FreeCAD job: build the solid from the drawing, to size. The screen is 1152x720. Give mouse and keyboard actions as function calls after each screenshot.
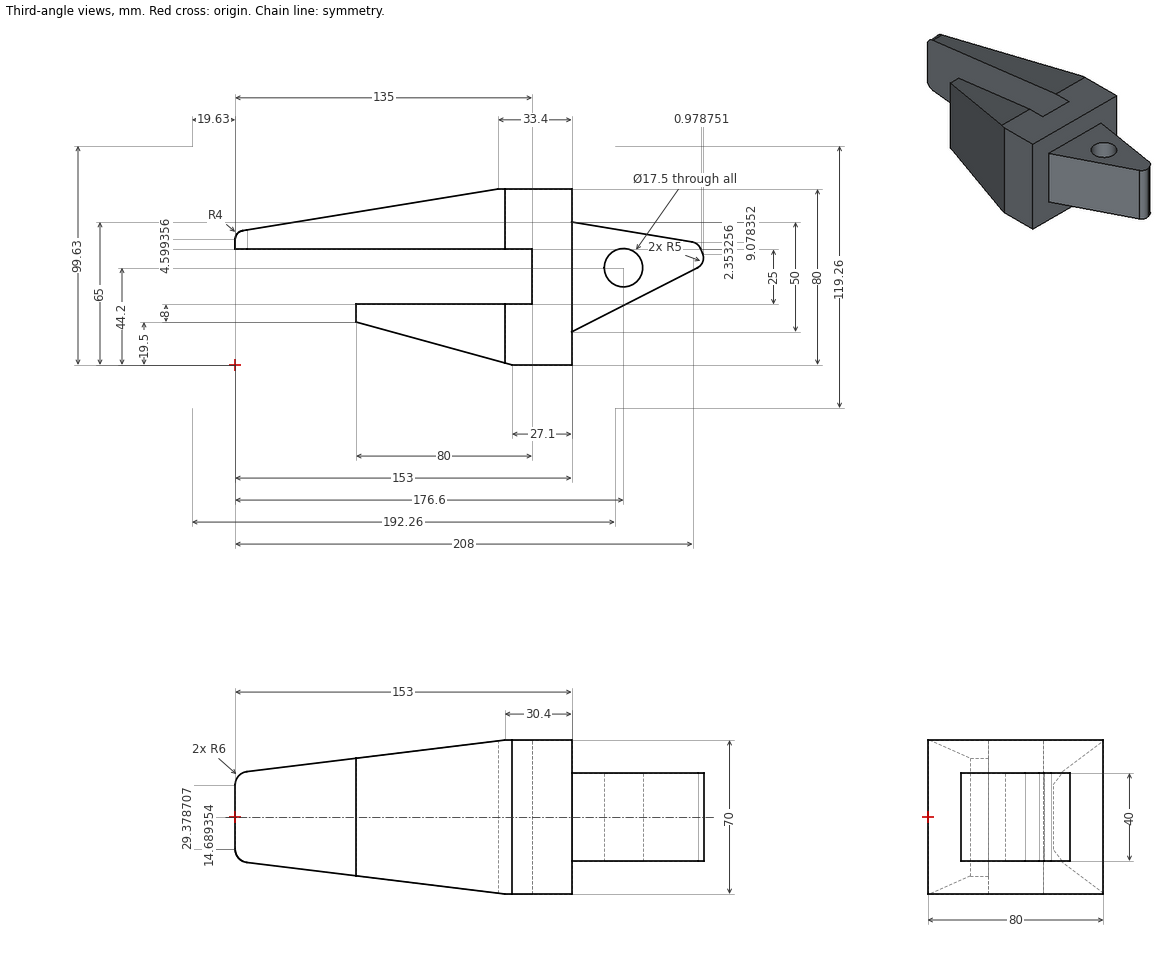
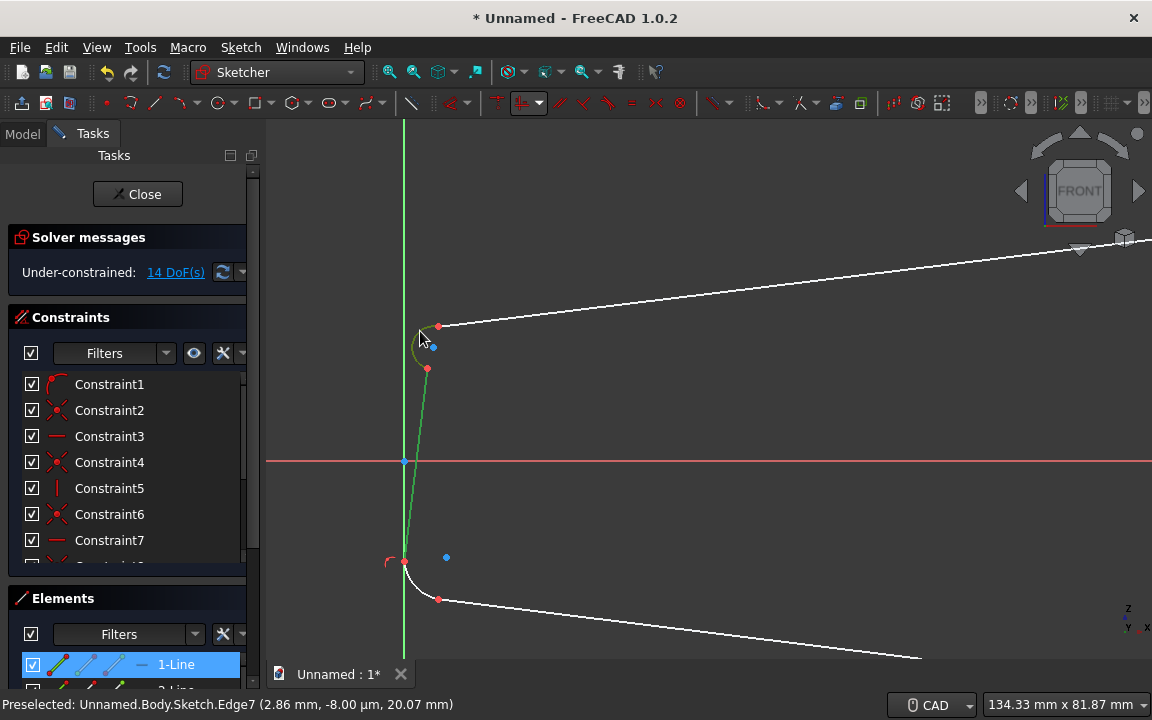
click(608, 104)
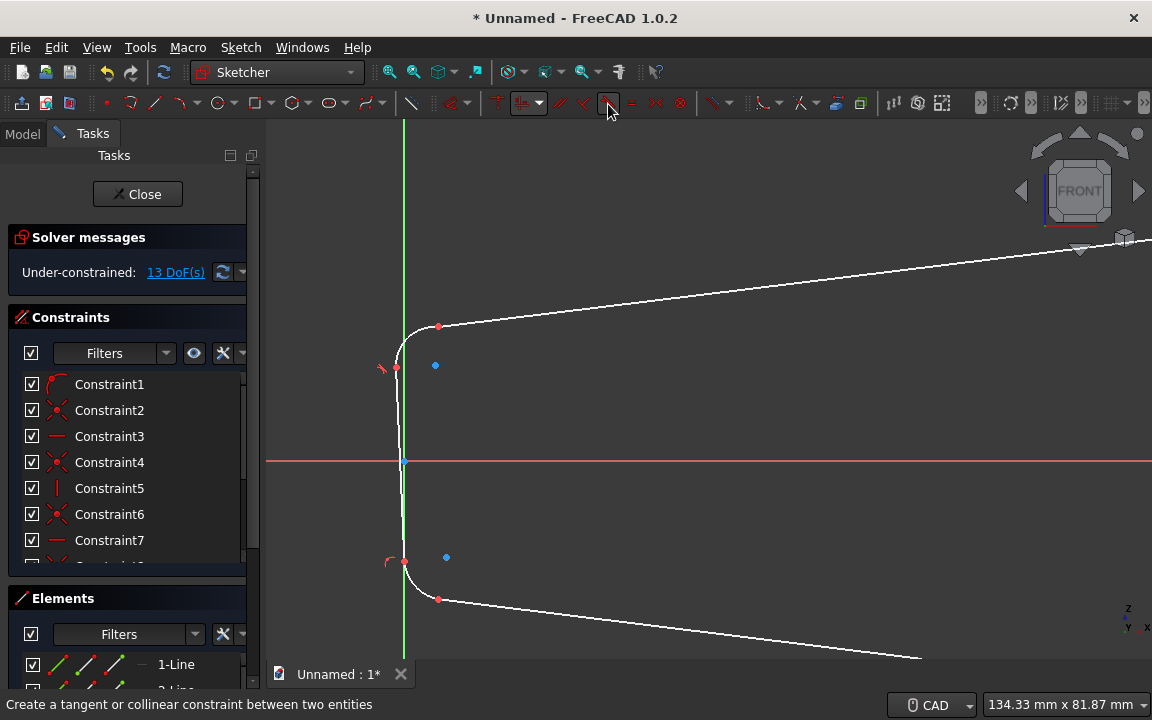
click(402, 503)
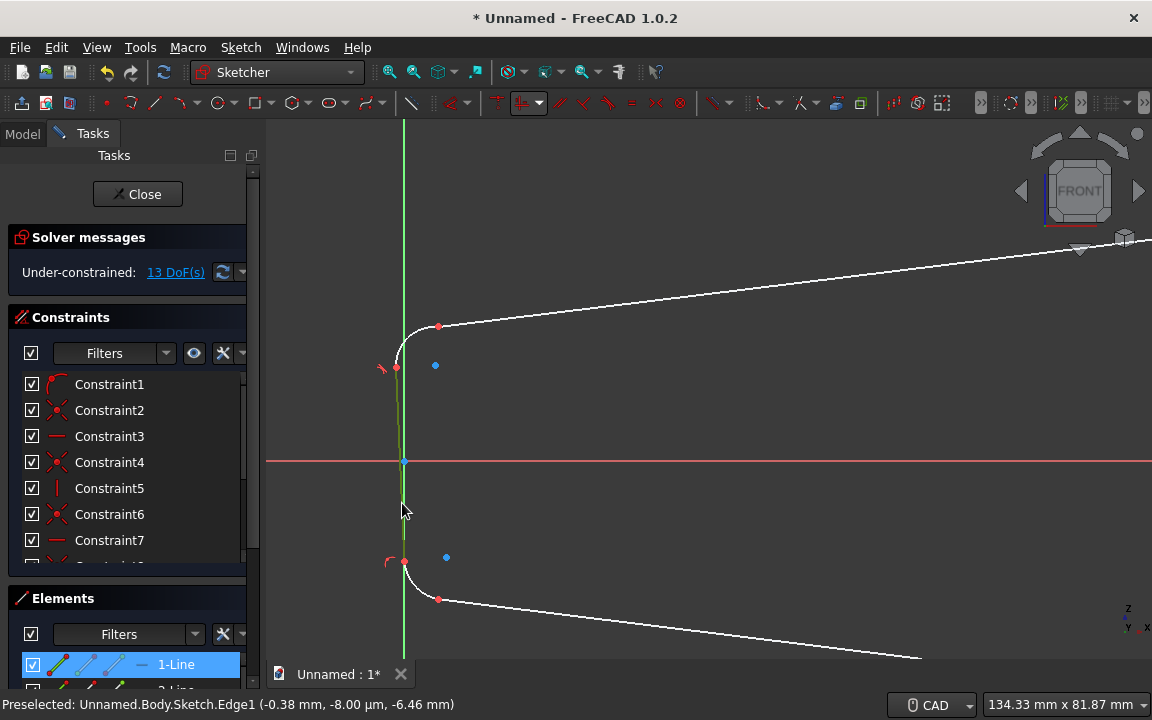
click(424, 593)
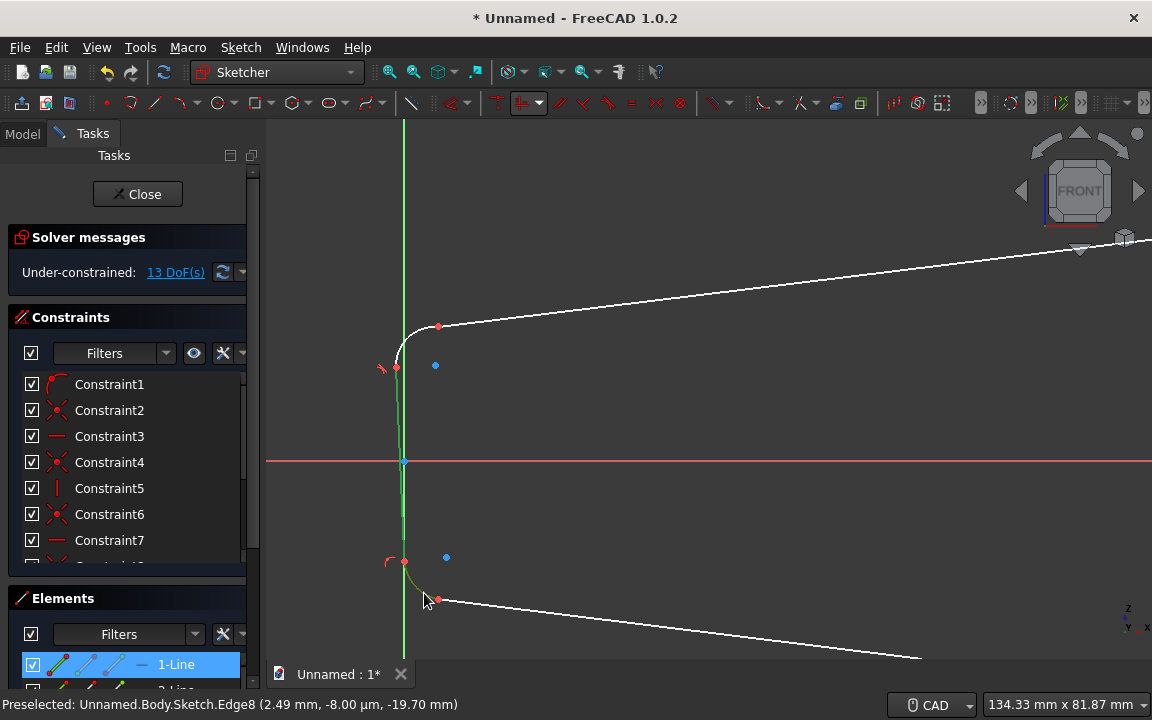
click(608, 104)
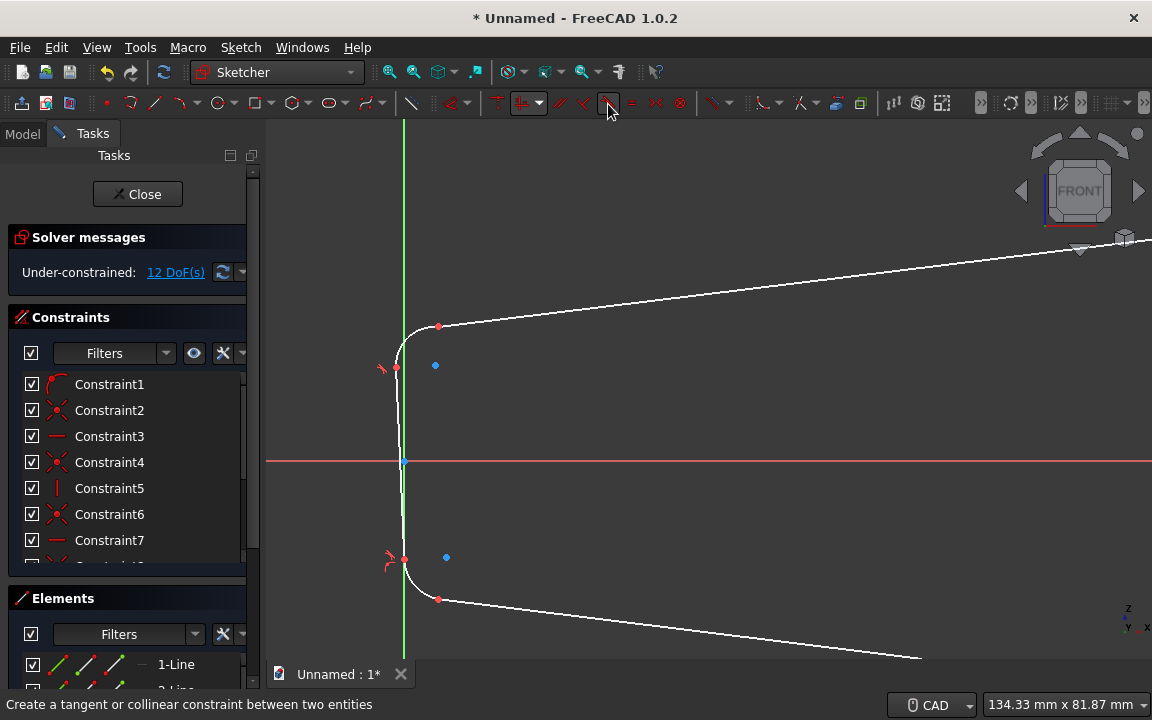
click(671, 299)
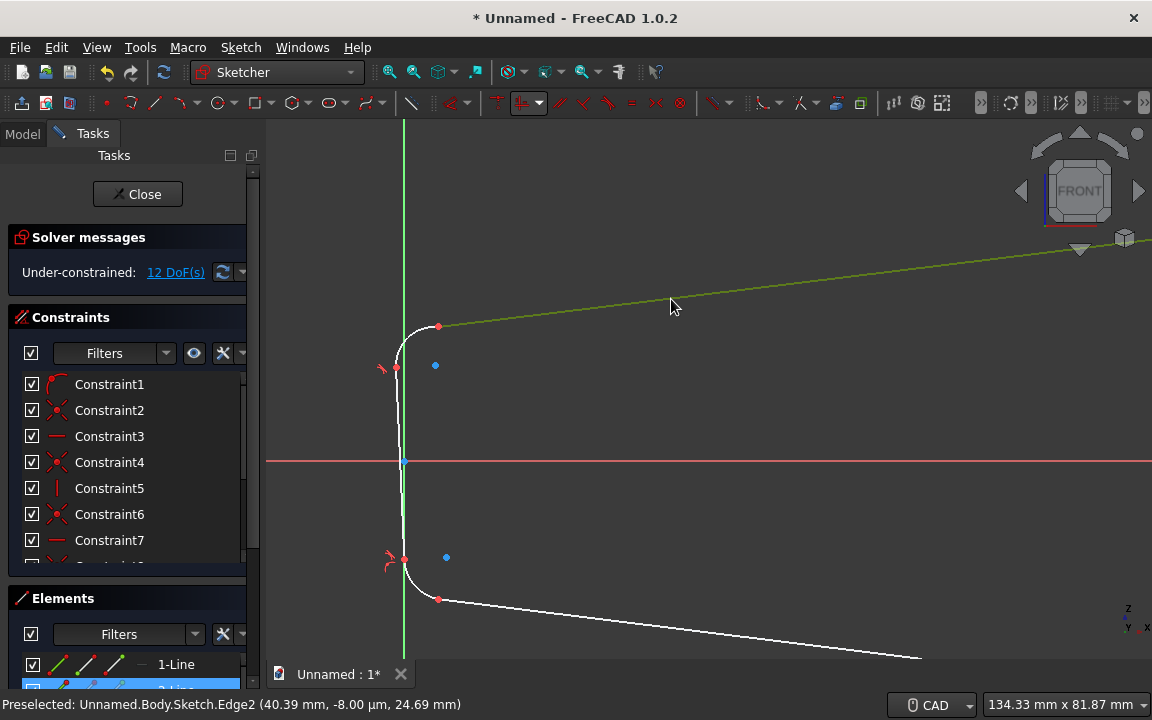
click(419, 330)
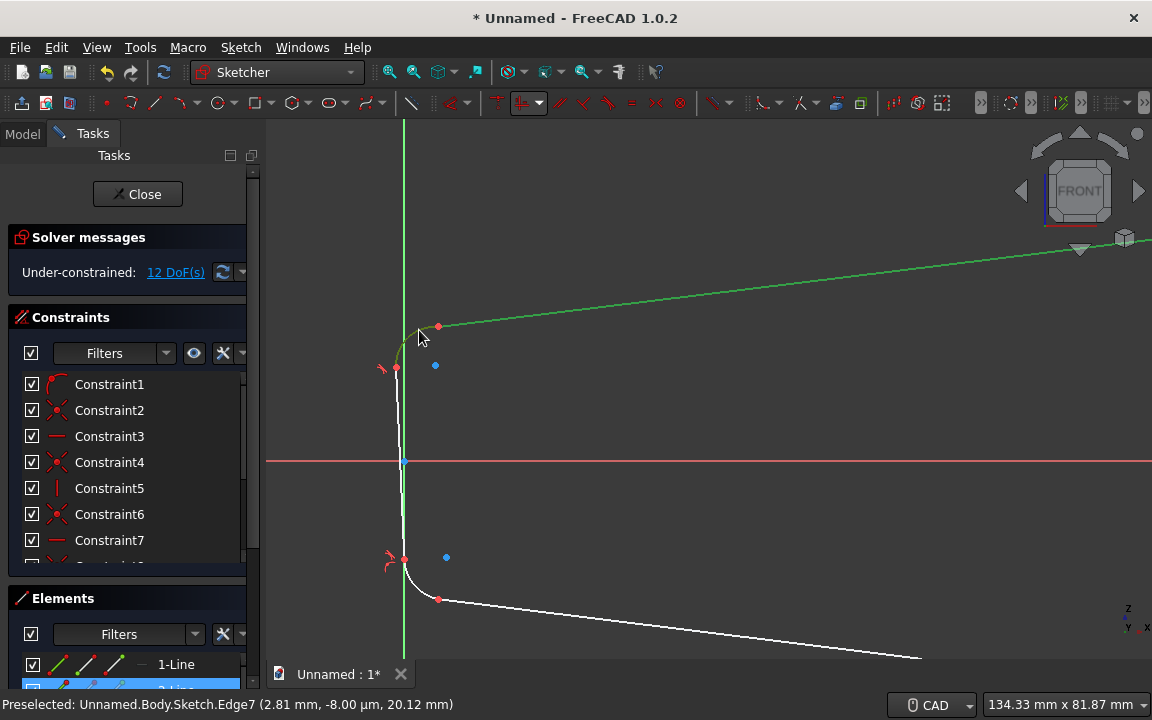
click(608, 104)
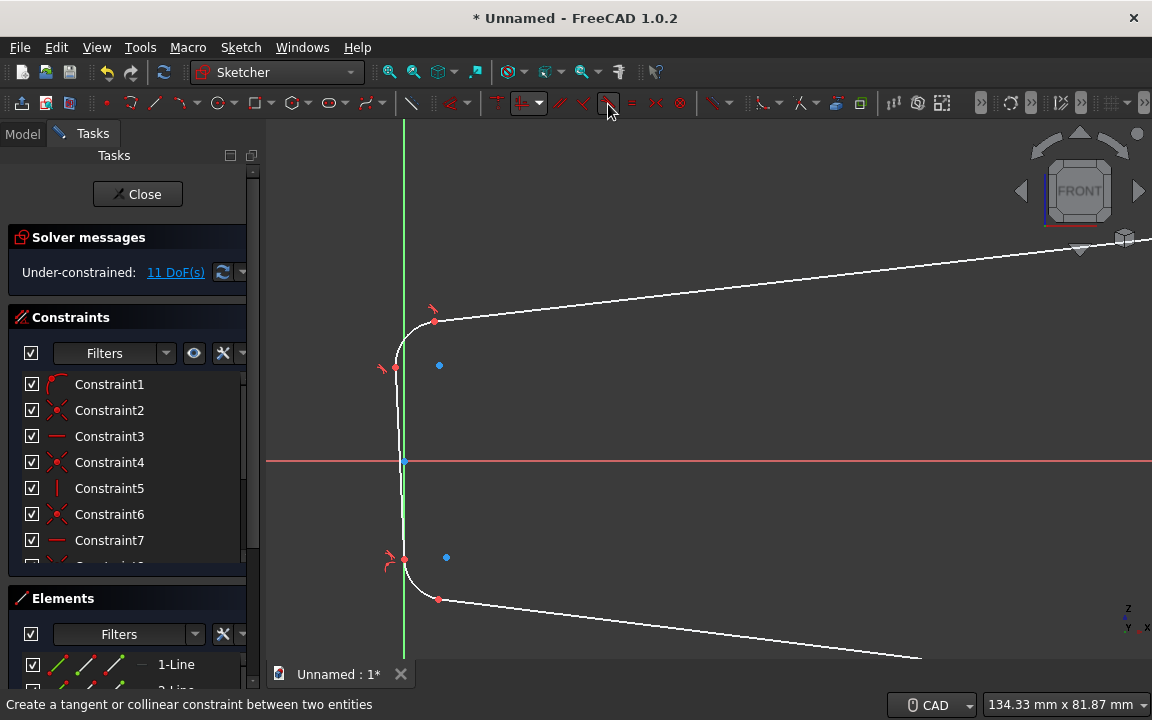
click(671, 628)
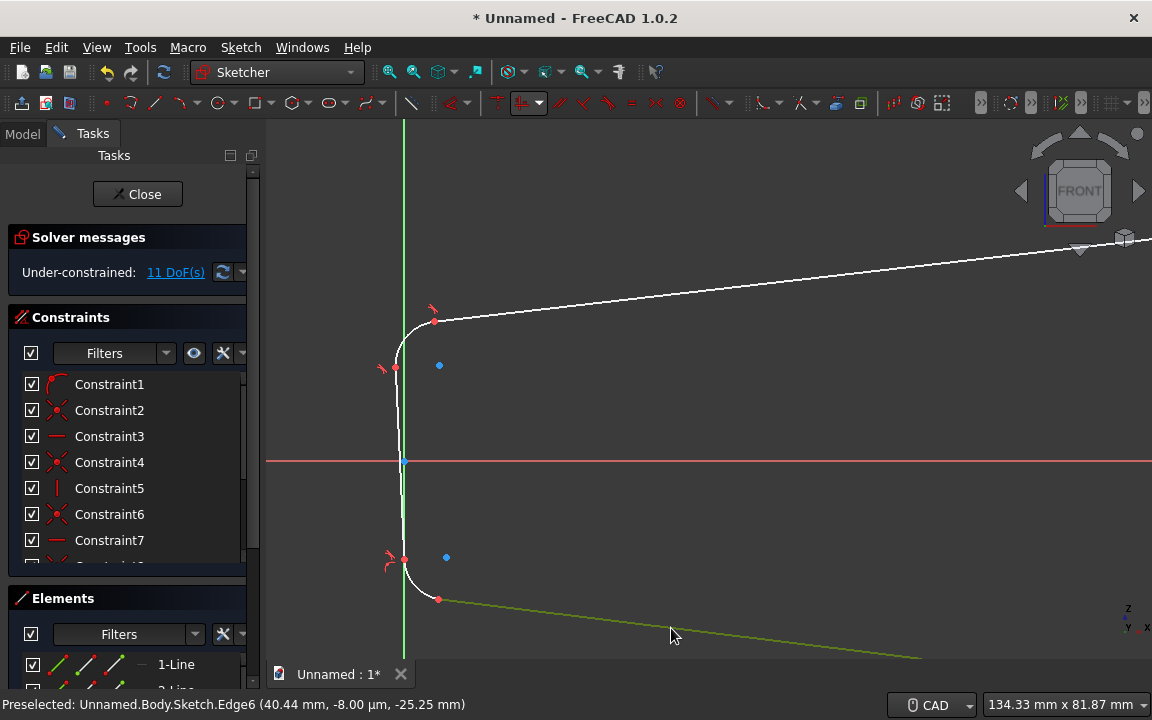
click(423, 593)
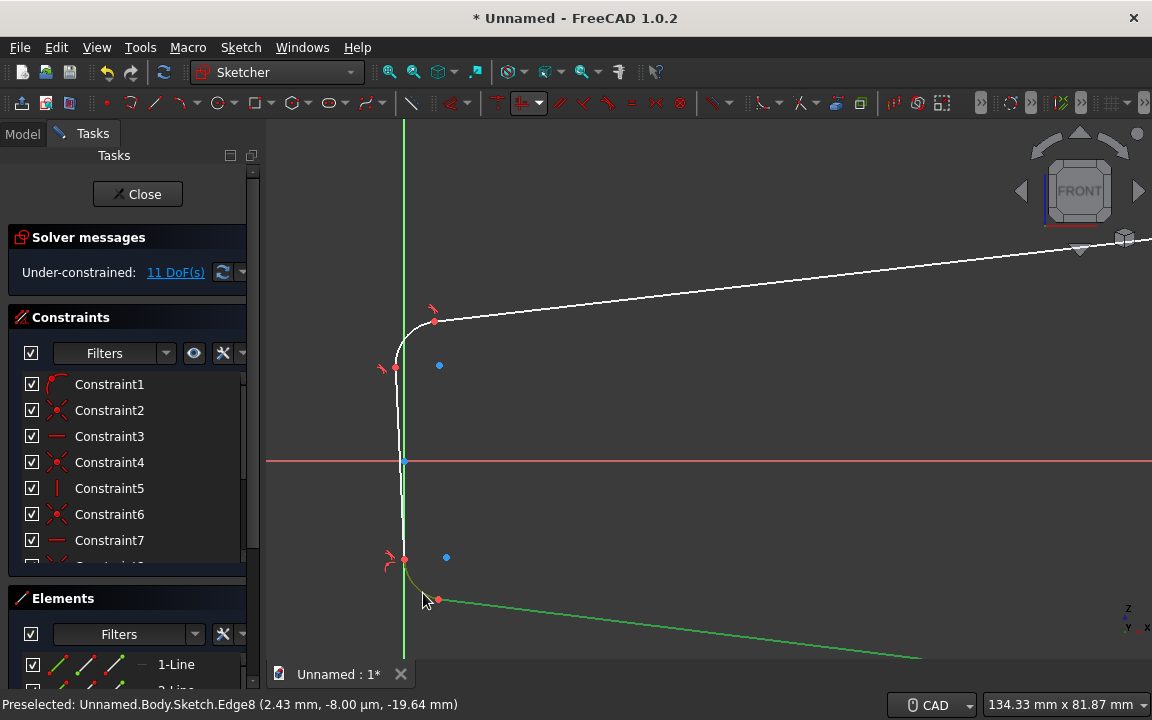
click(608, 104)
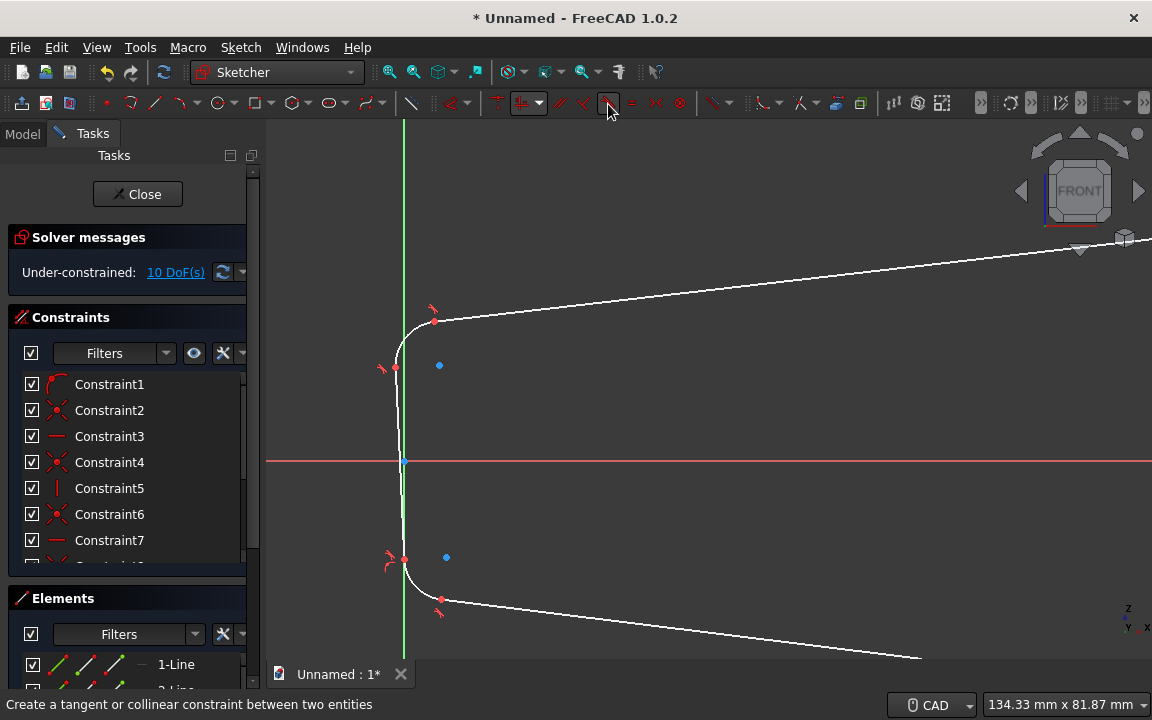
click(402, 502)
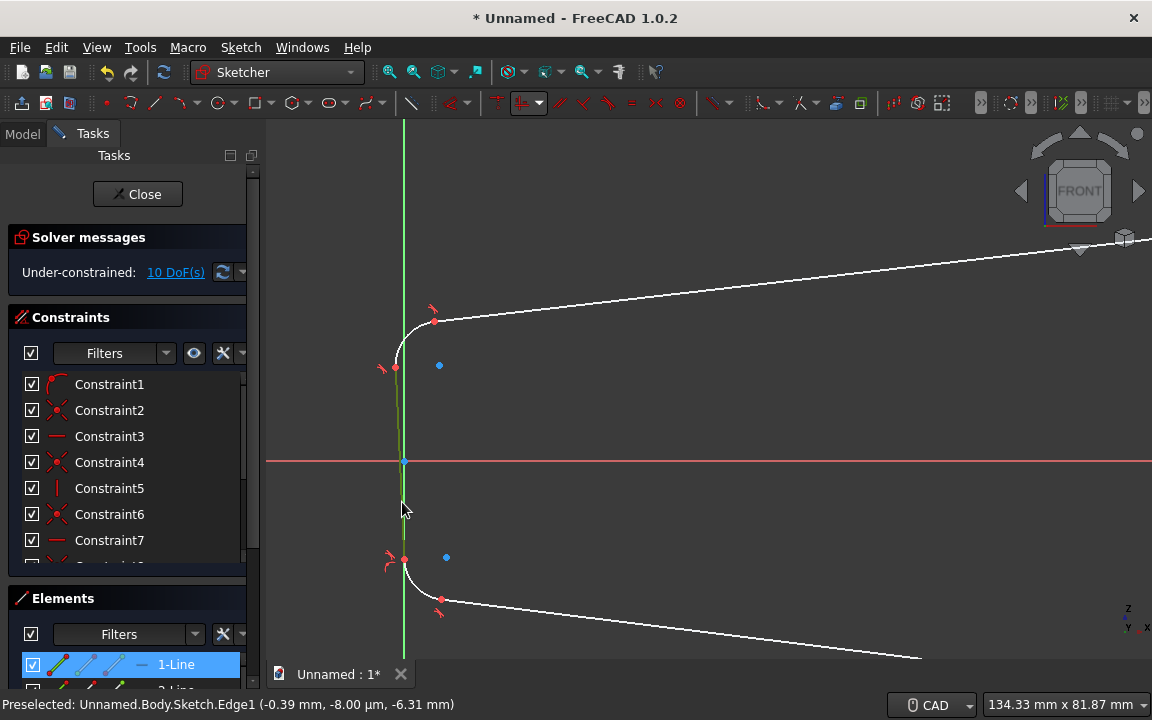
key(v)